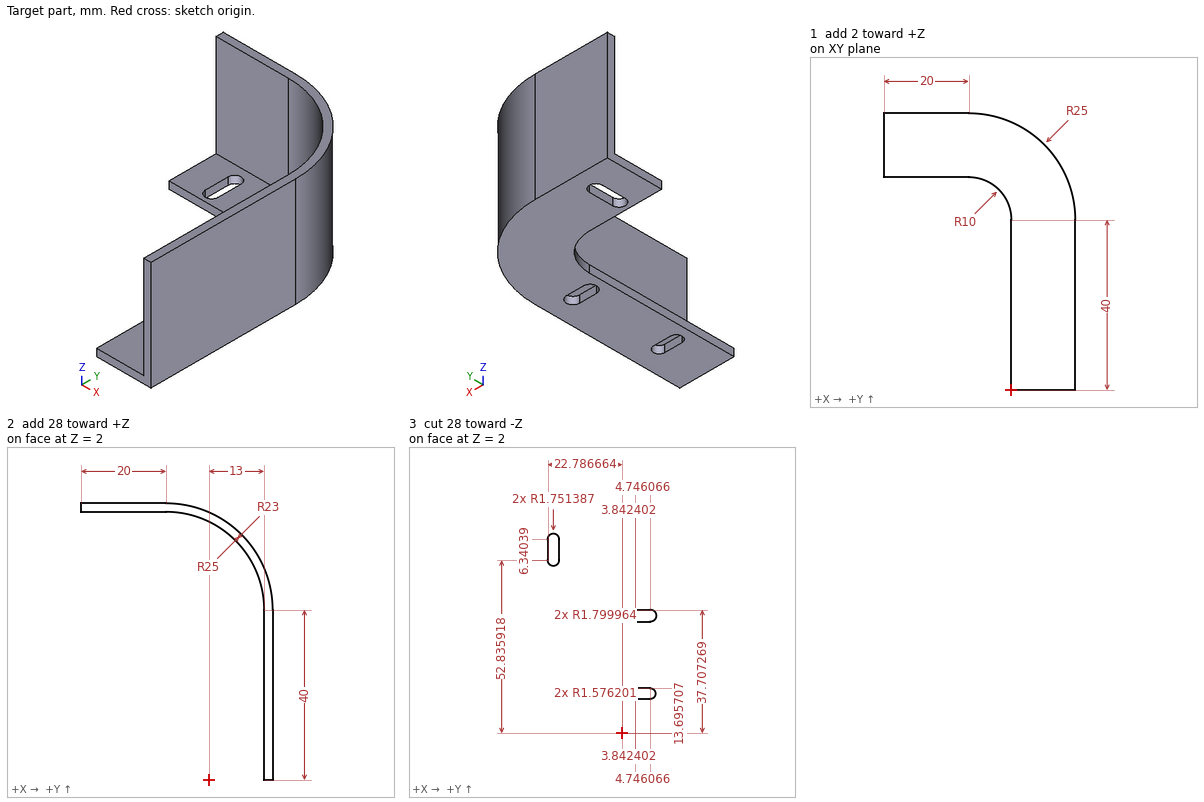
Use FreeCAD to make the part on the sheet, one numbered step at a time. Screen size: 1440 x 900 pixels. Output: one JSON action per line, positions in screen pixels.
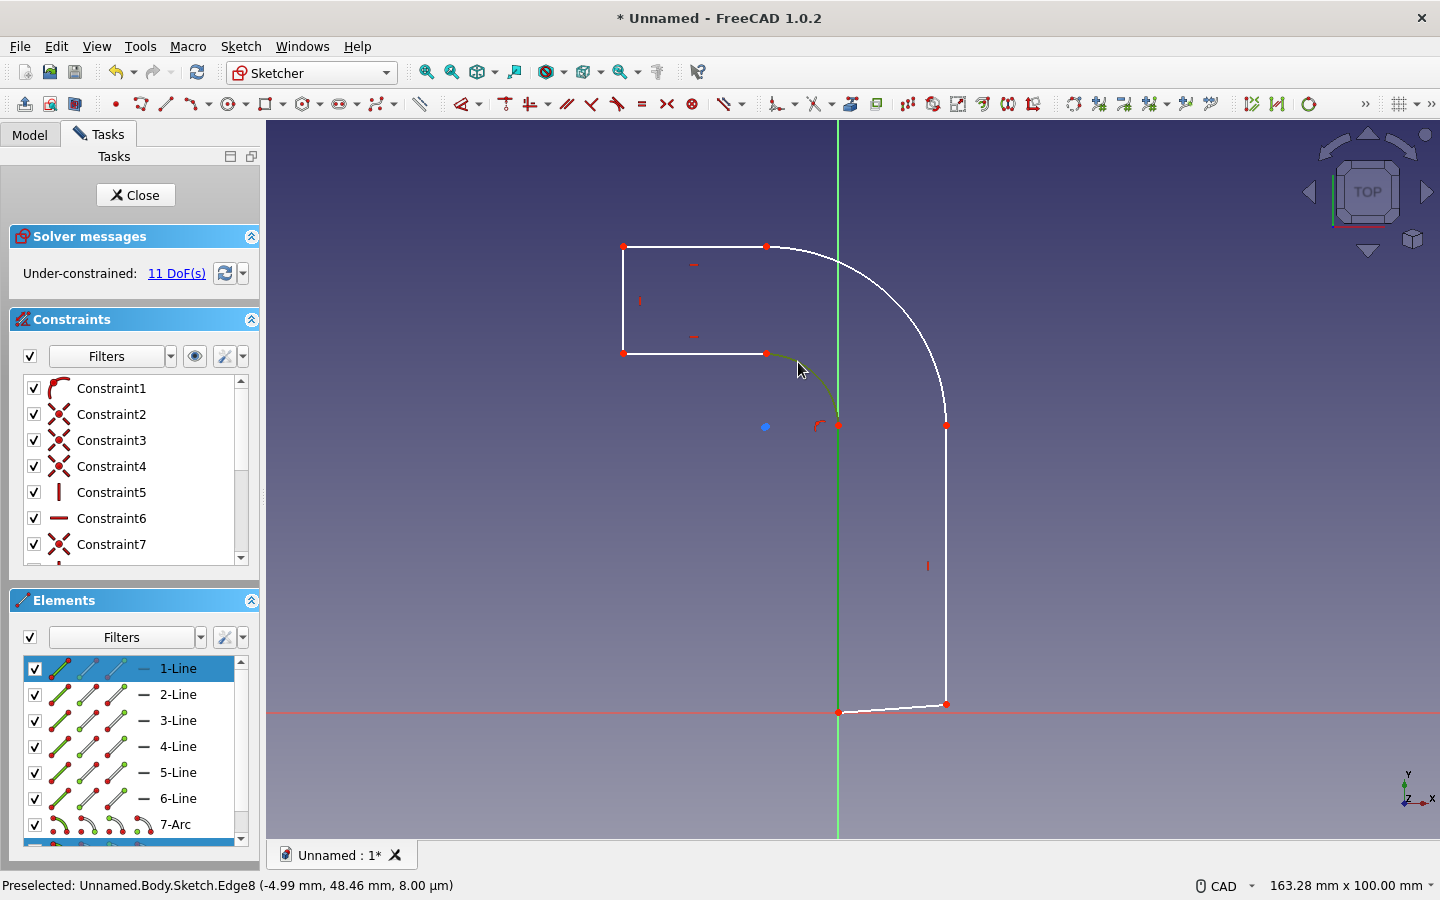
{"action": "left_click", "coordinate": [617, 104]}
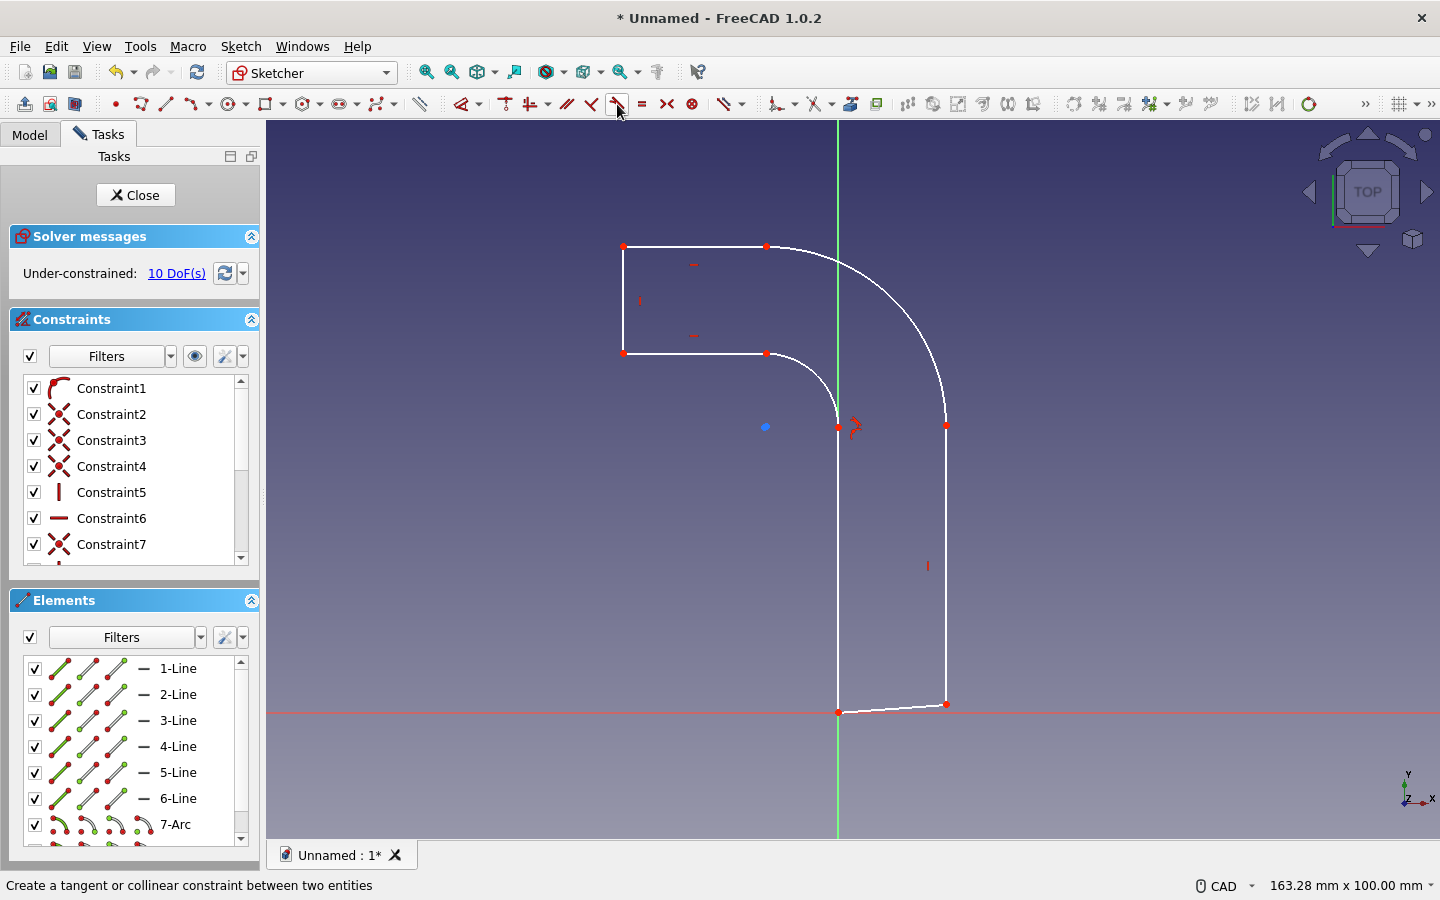
{"action": "left_click", "coordinate": [946, 621]}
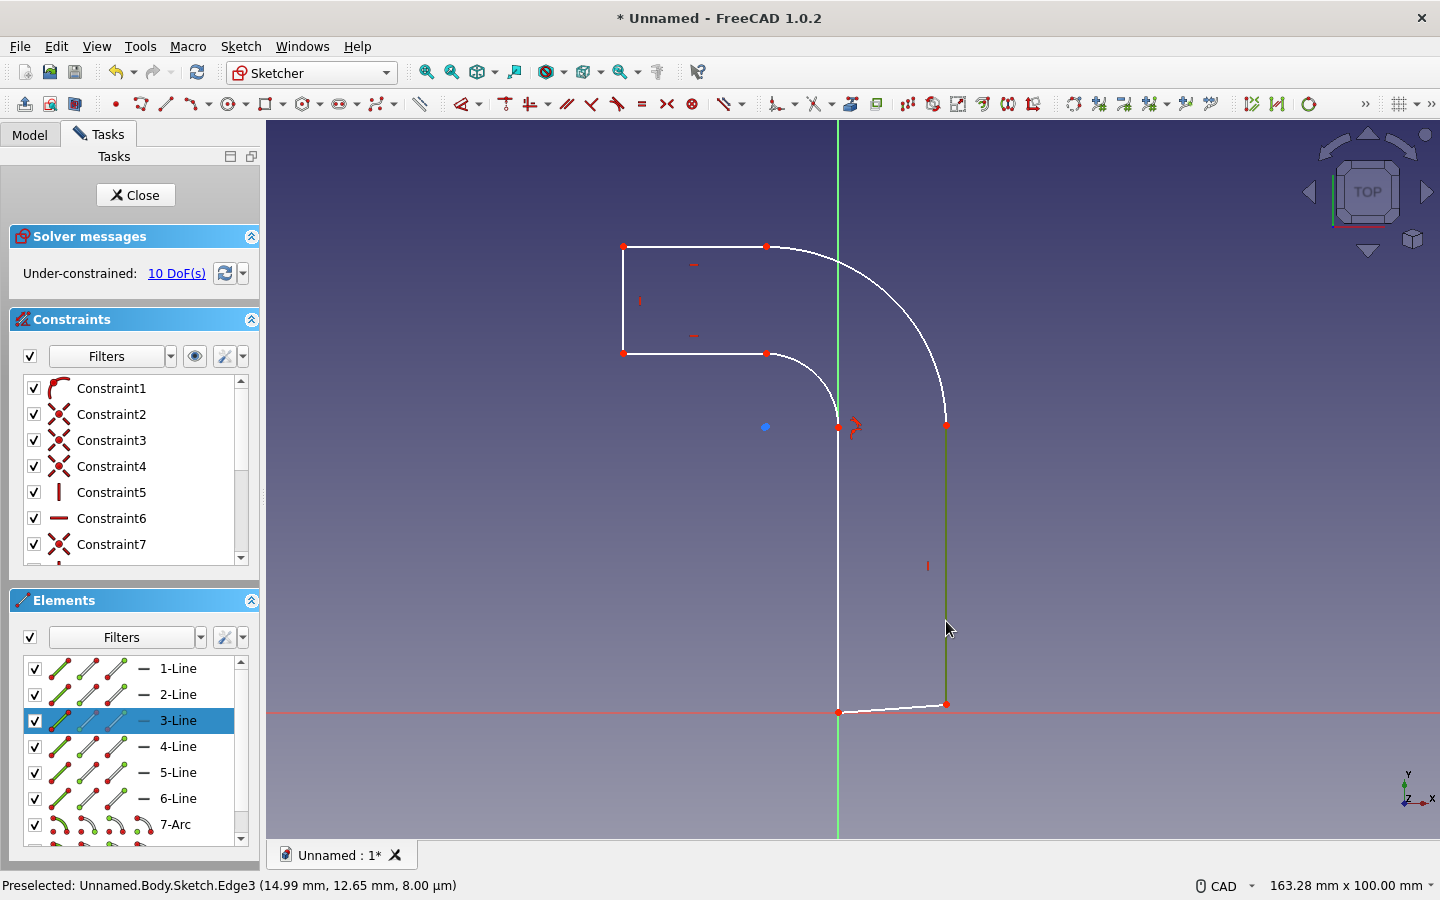
{"action": "left_click", "coordinate": [926, 345]}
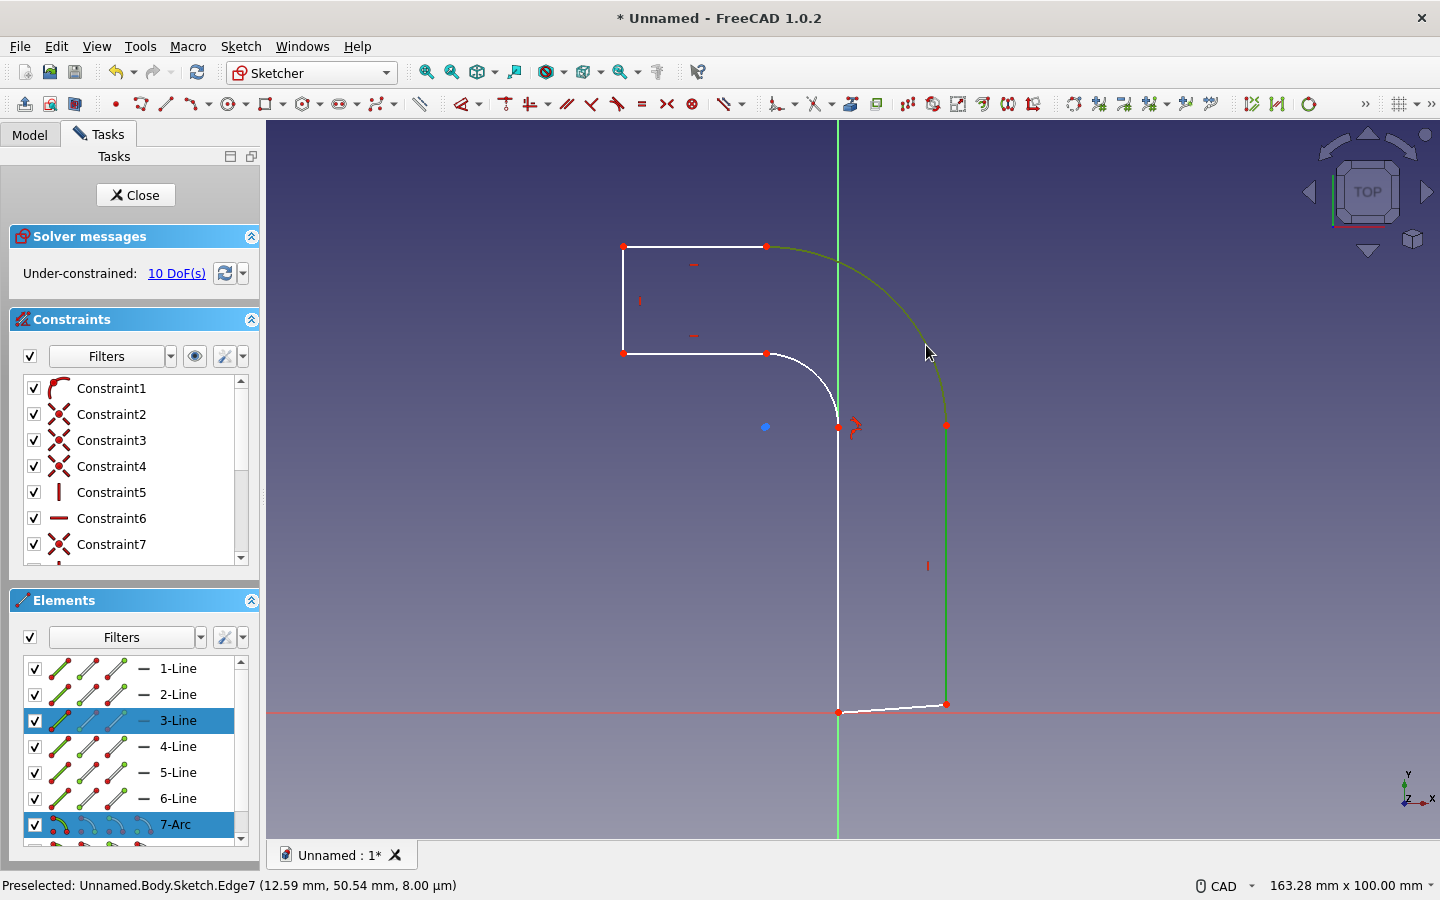
{"action": "left_click", "coordinate": [617, 104]}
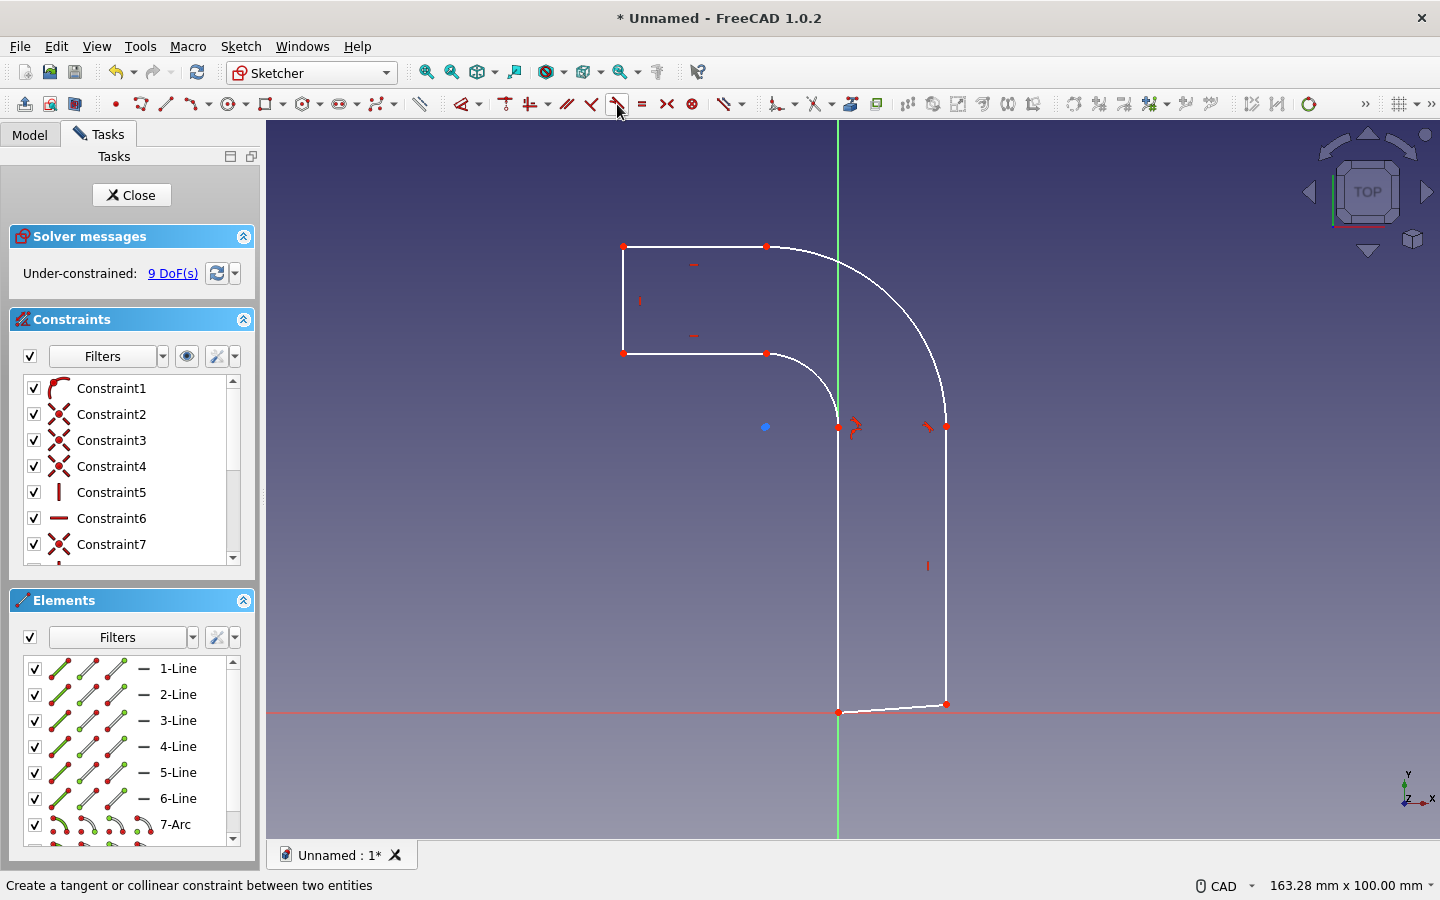
{"action": "left_click", "coordinate": [723, 247]}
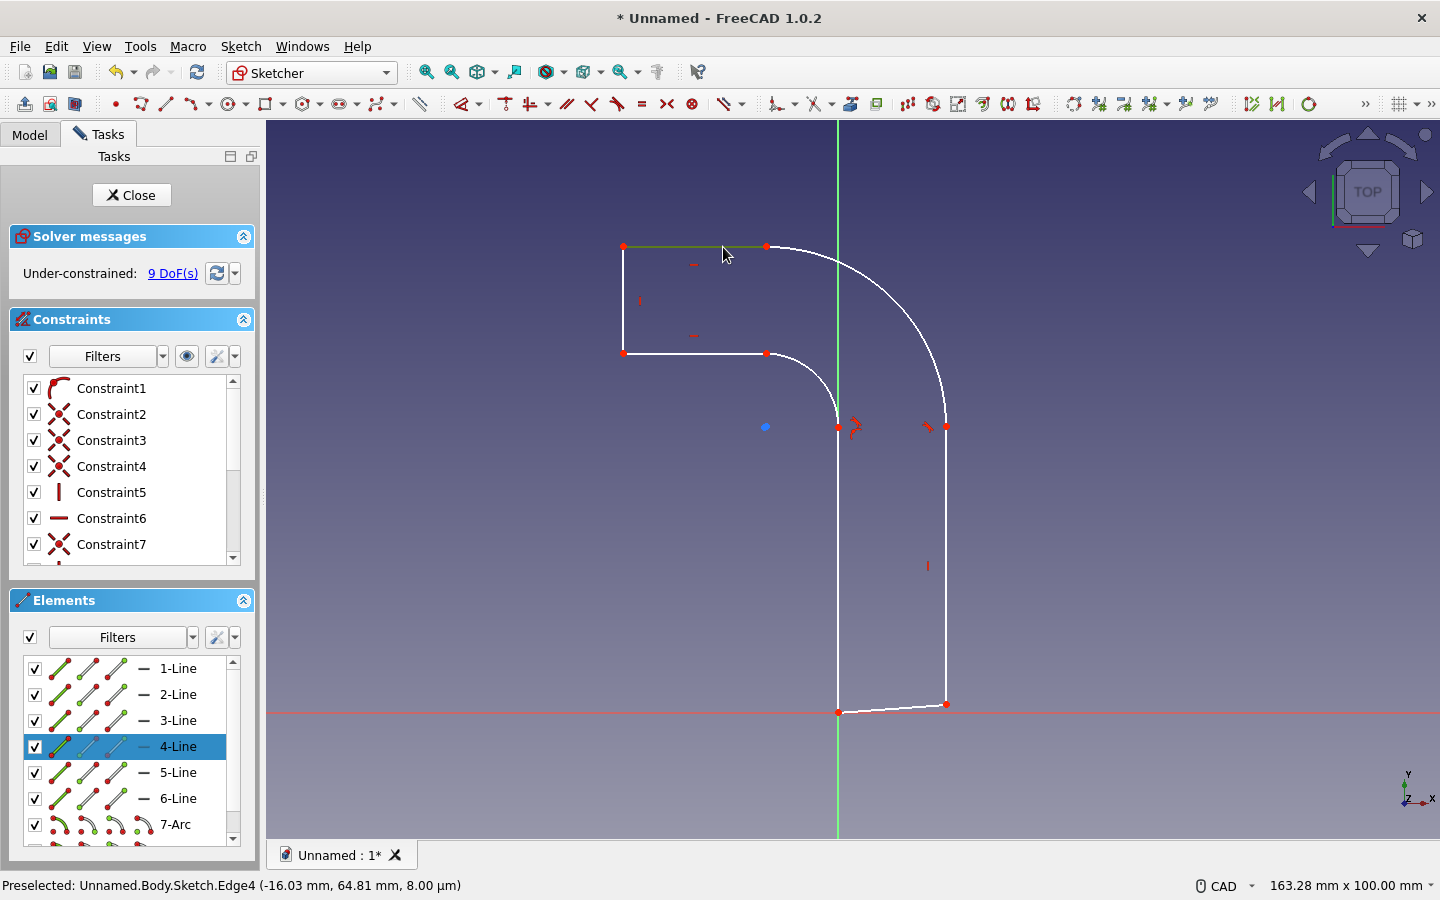
{"action": "left_click", "coordinate": [926, 345]}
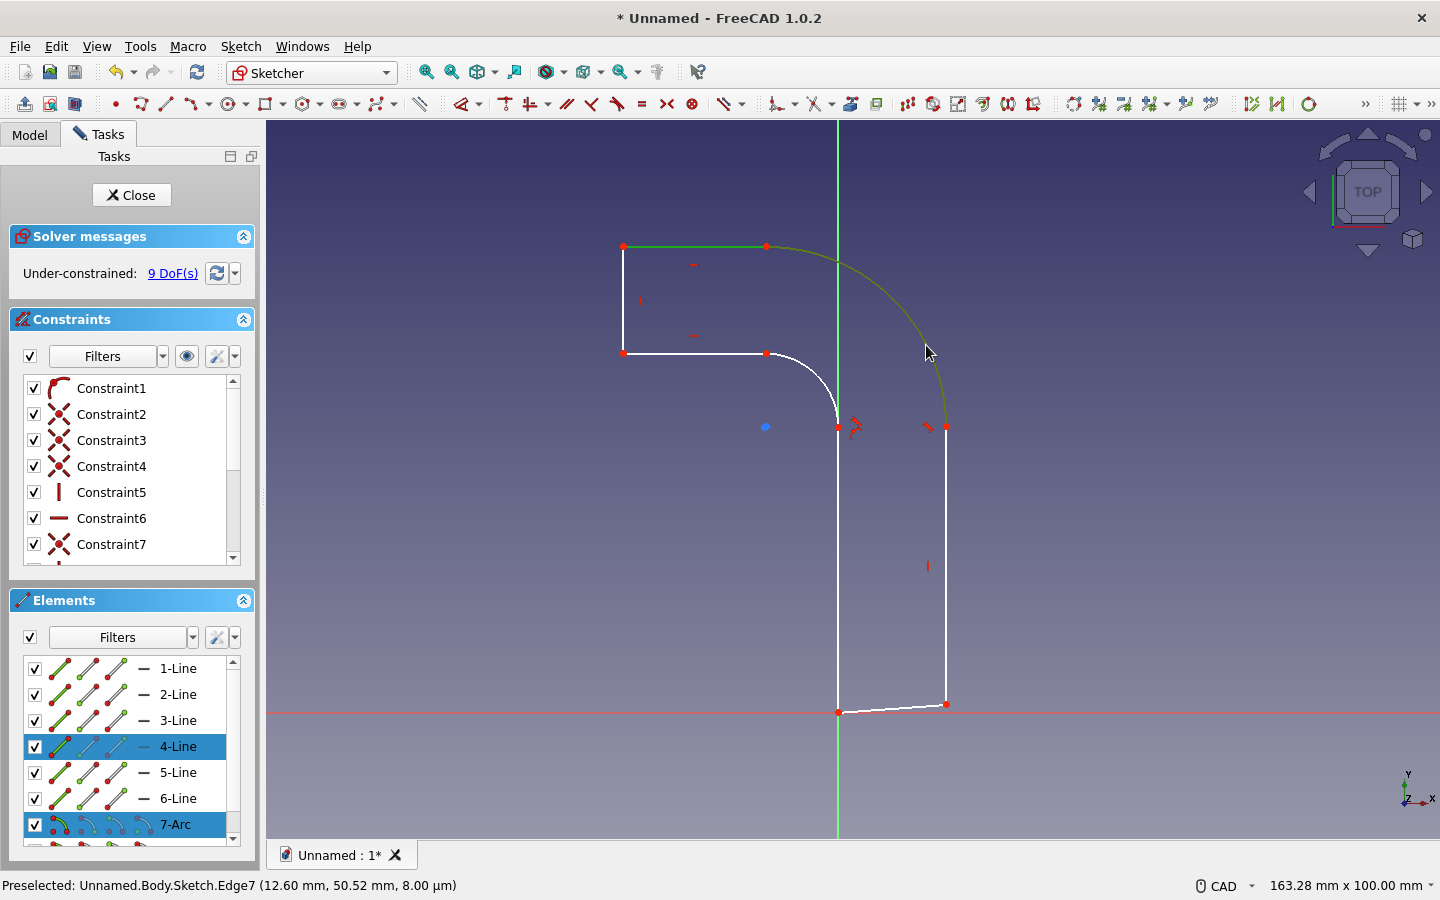
{"action": "left_click", "coordinate": [617, 104]}